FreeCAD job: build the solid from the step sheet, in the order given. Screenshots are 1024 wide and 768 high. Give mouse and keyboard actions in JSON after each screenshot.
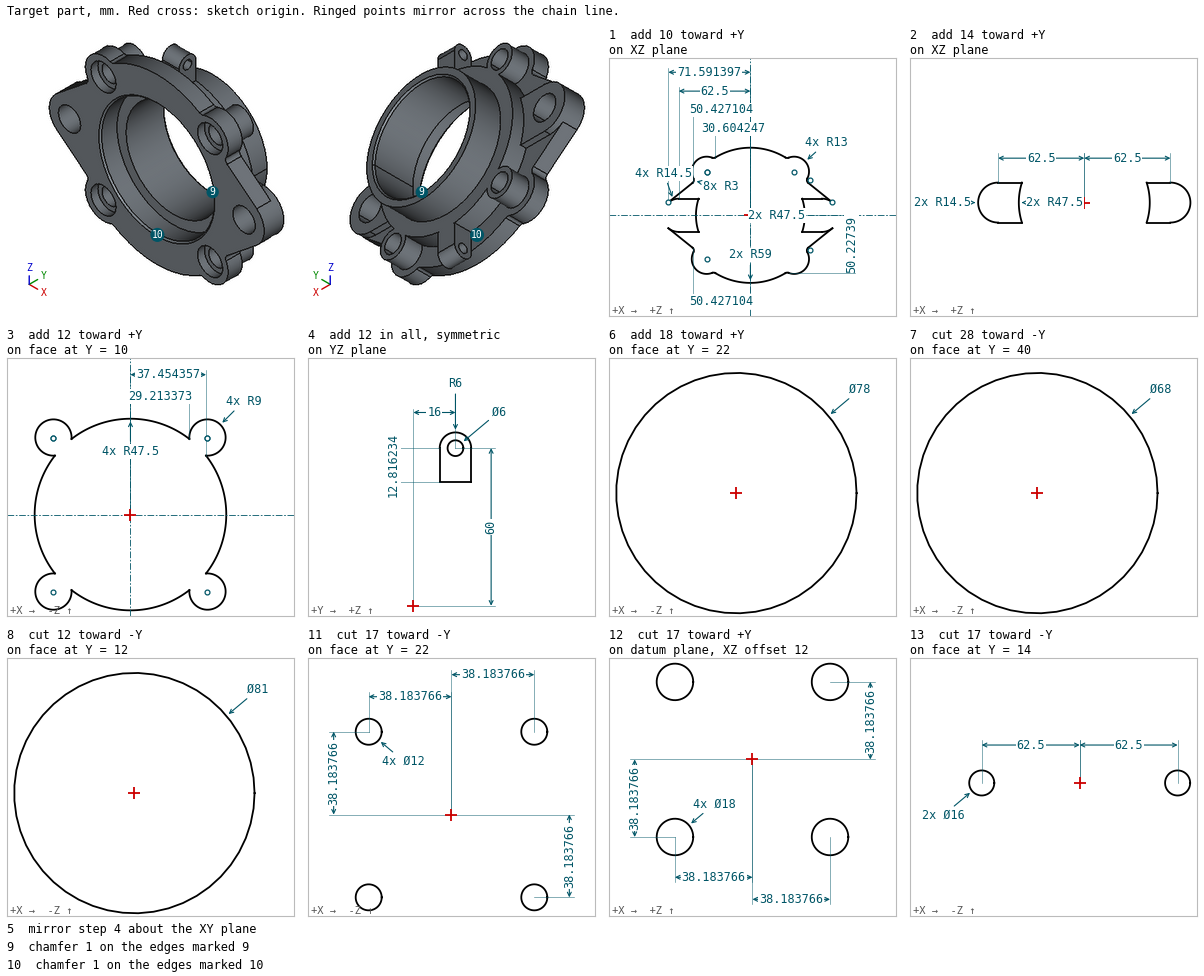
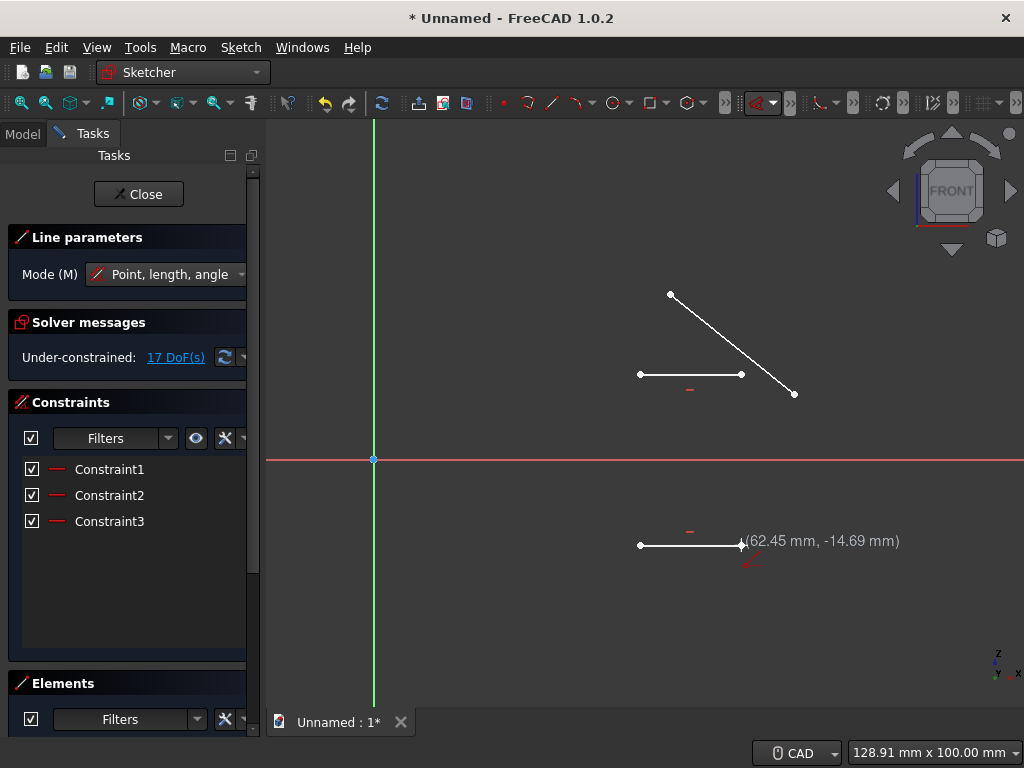
{"action": "left_click", "coordinate": [795, 526]}
{"action": "left_click", "coordinate": [670, 626]}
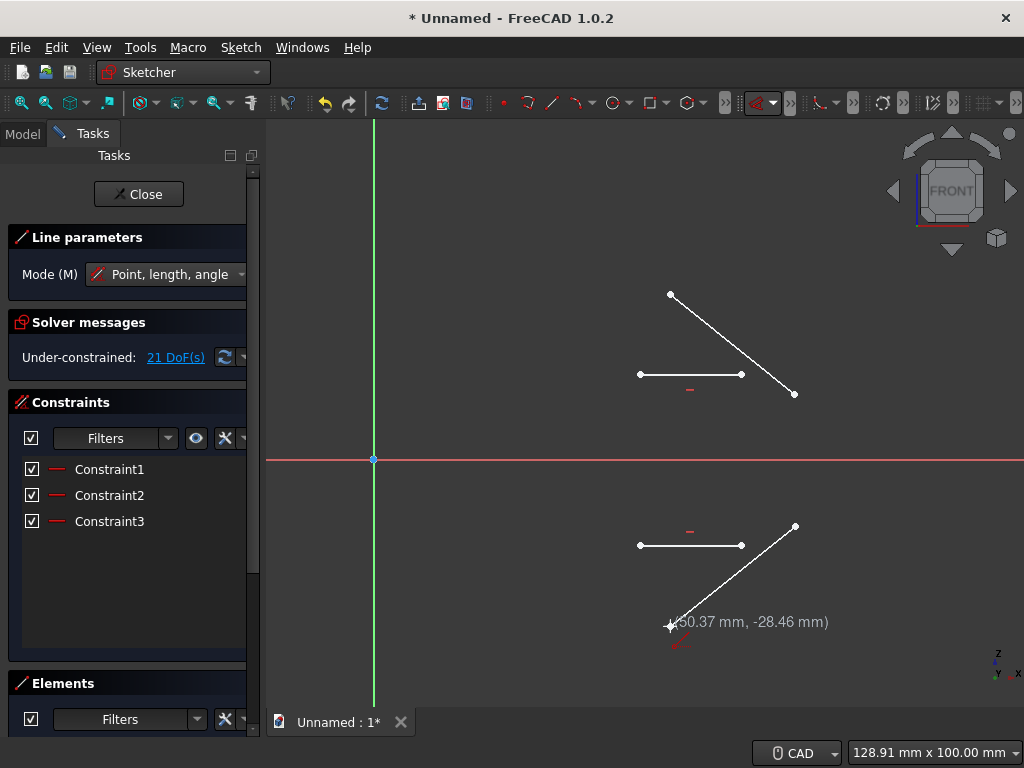
{"action": "scroll", "coordinate": [742, 375], "scroll_direction": "down", "scroll_amount": 4}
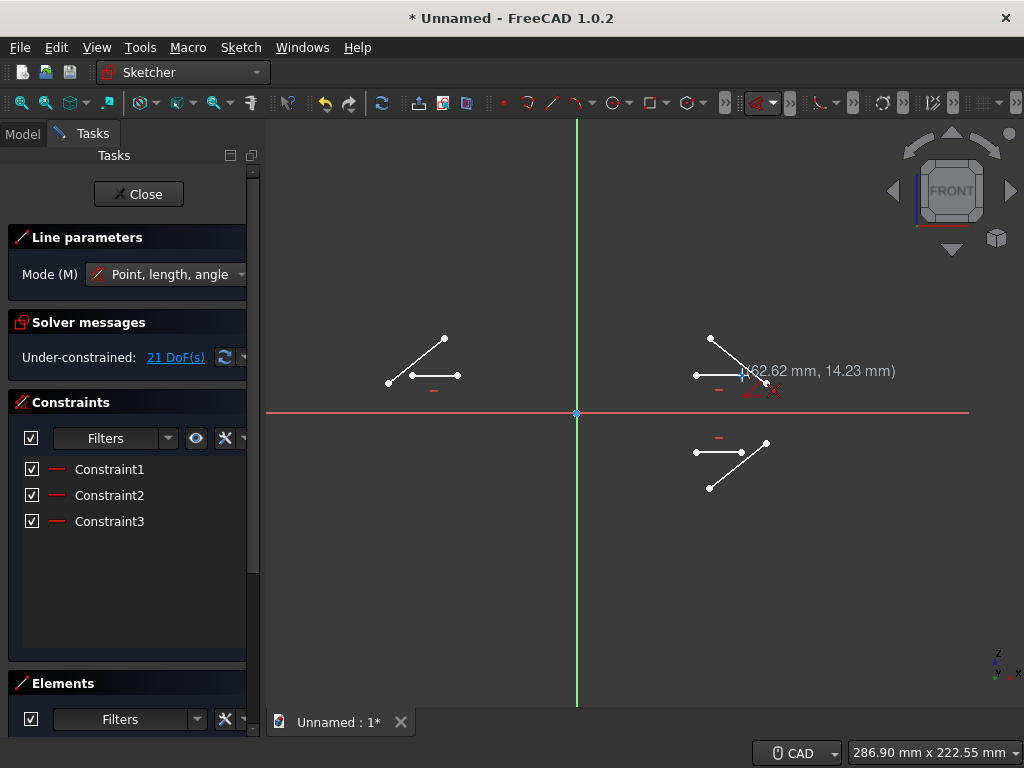
{"action": "left_click", "coordinate": [444, 488]}
{"action": "left_click", "coordinate": [388, 443]}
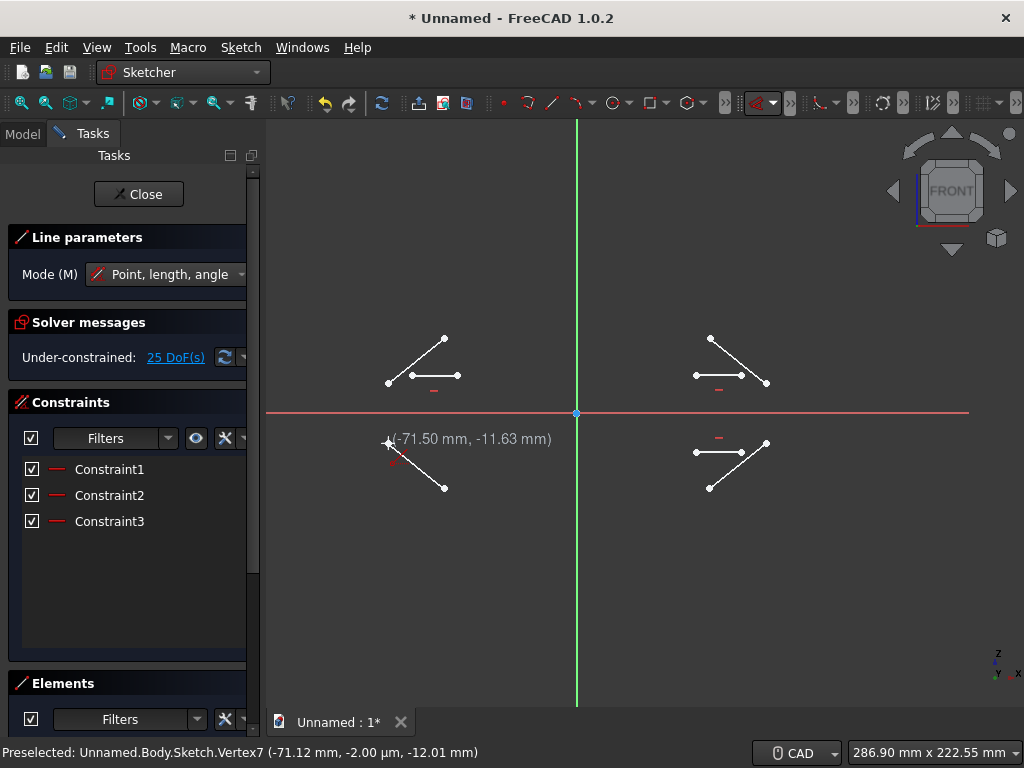
{"action": "scroll", "coordinate": [412, 452], "scroll_direction": "up", "scroll_amount": 4}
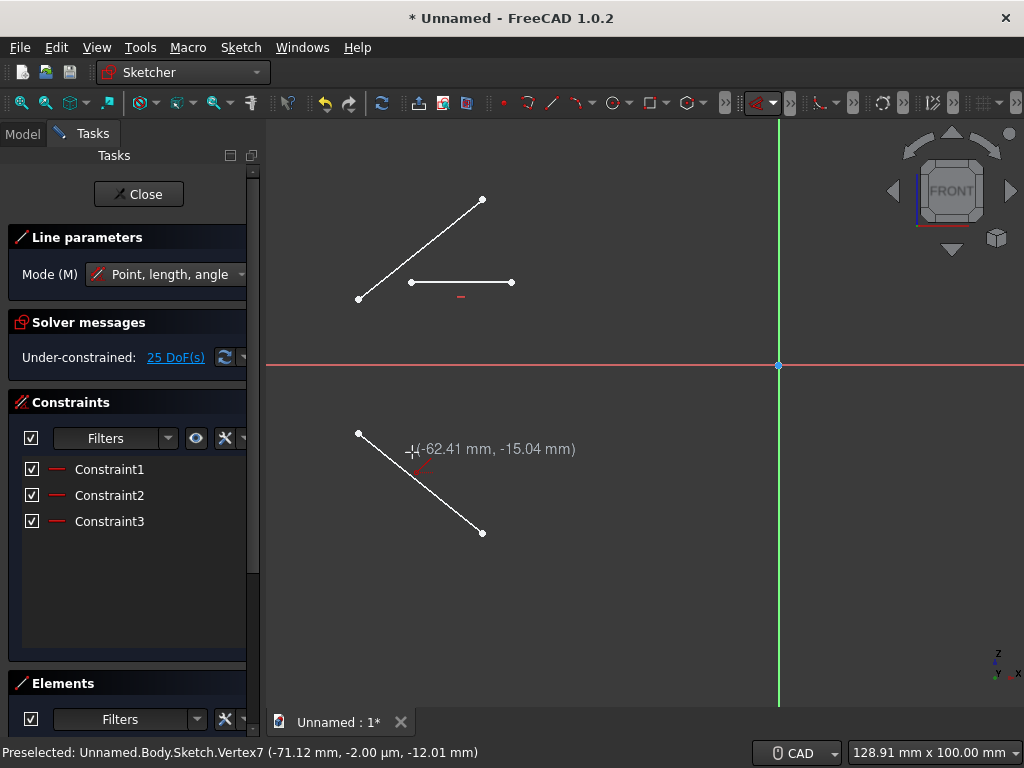
{"action": "left_click", "coordinate": [411, 450]}
{"action": "left_click", "coordinate": [513, 450]}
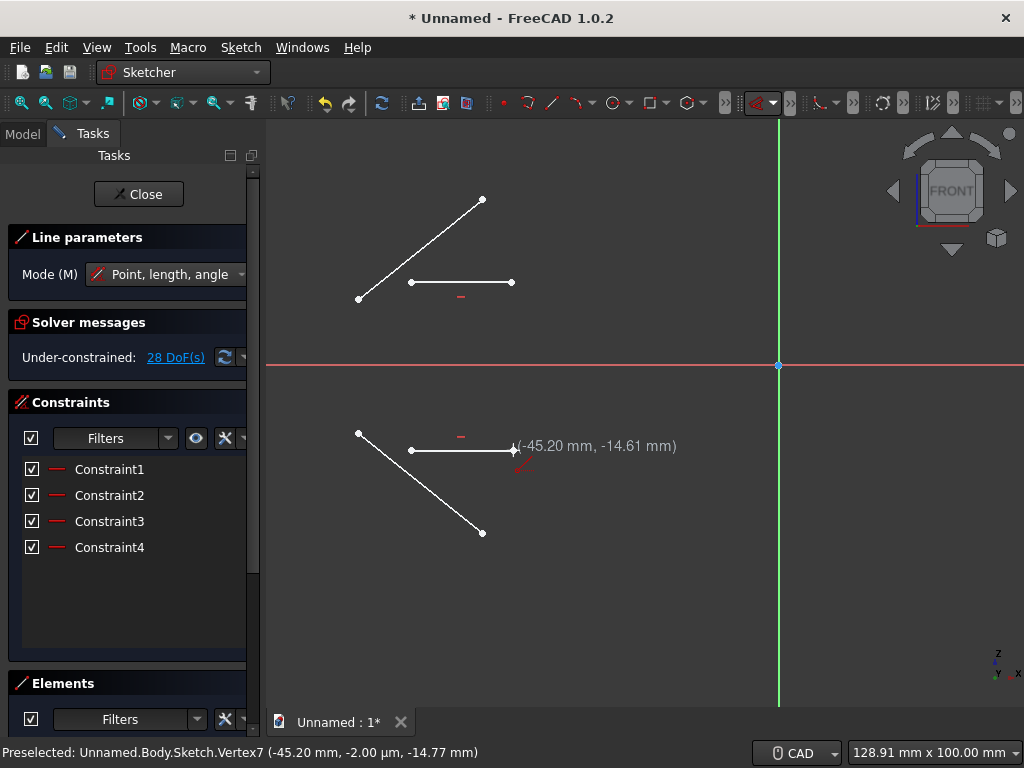
{"action": "key", "text": "g 3 a"}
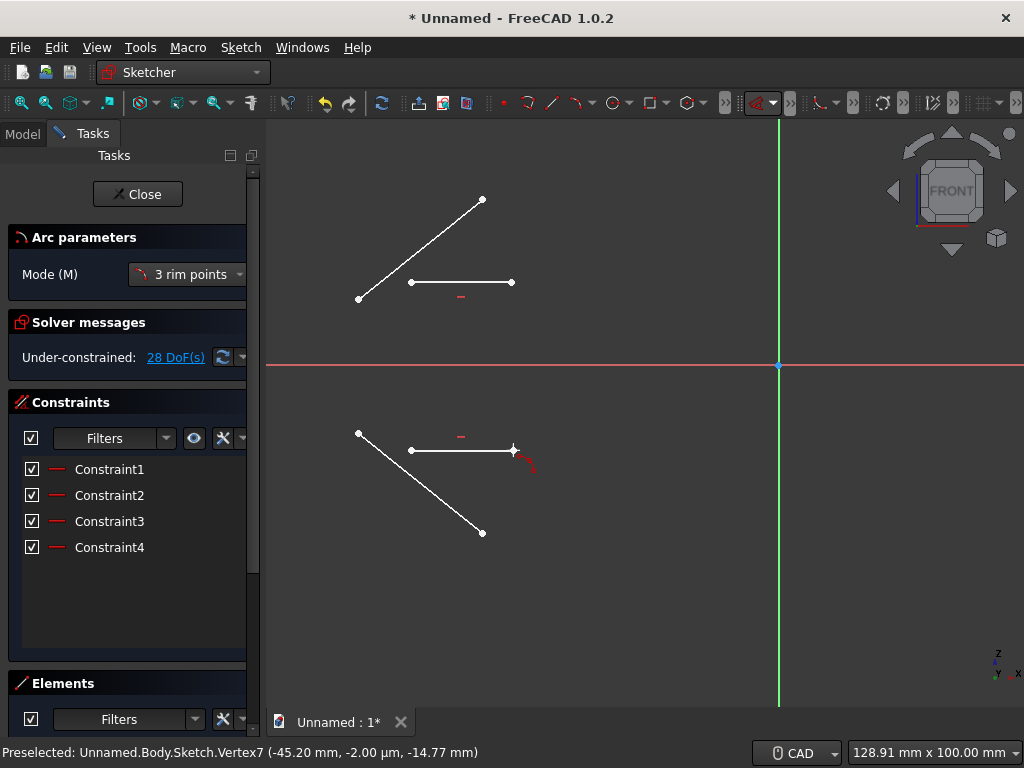
{"action": "left_click", "coordinate": [412, 282]}
{"action": "left_click", "coordinate": [358, 300]}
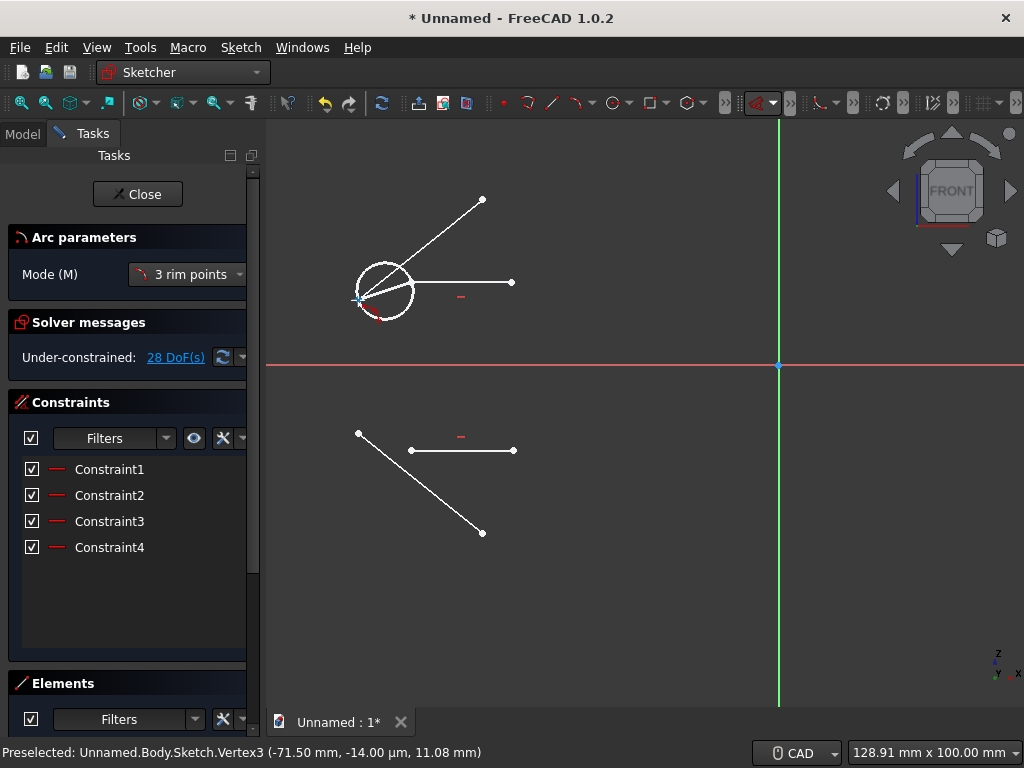
{"action": "scroll", "coordinate": [383, 285], "scroll_direction": "up", "scroll_amount": 6}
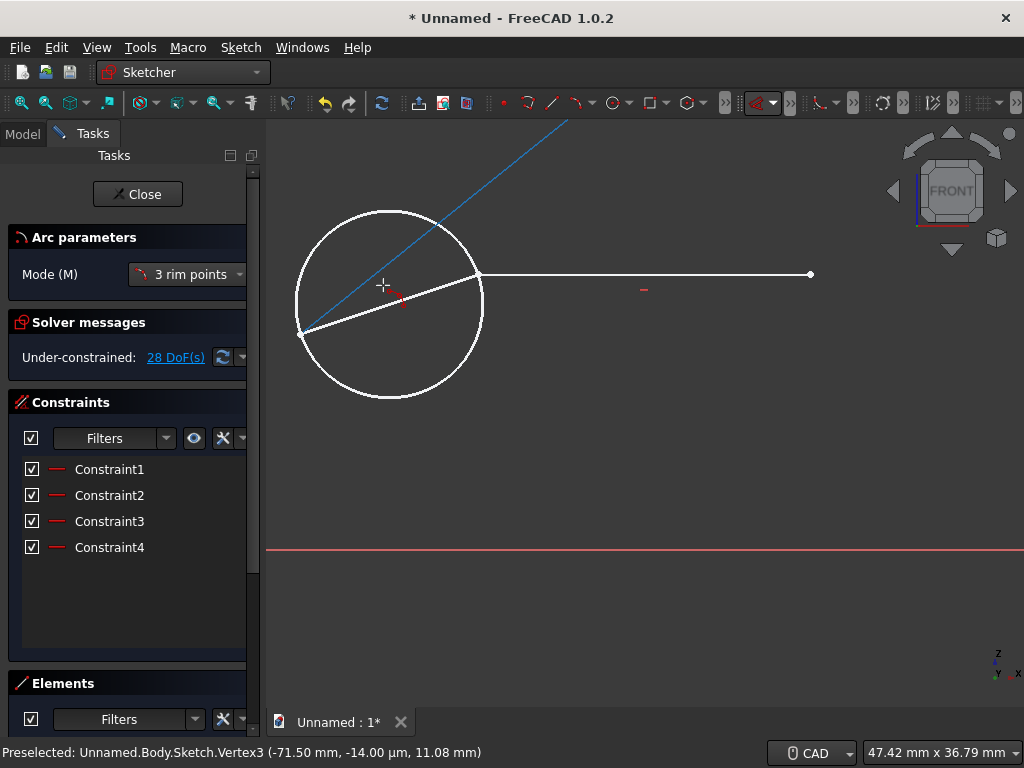
{"action": "left_click", "coordinate": [382, 283]}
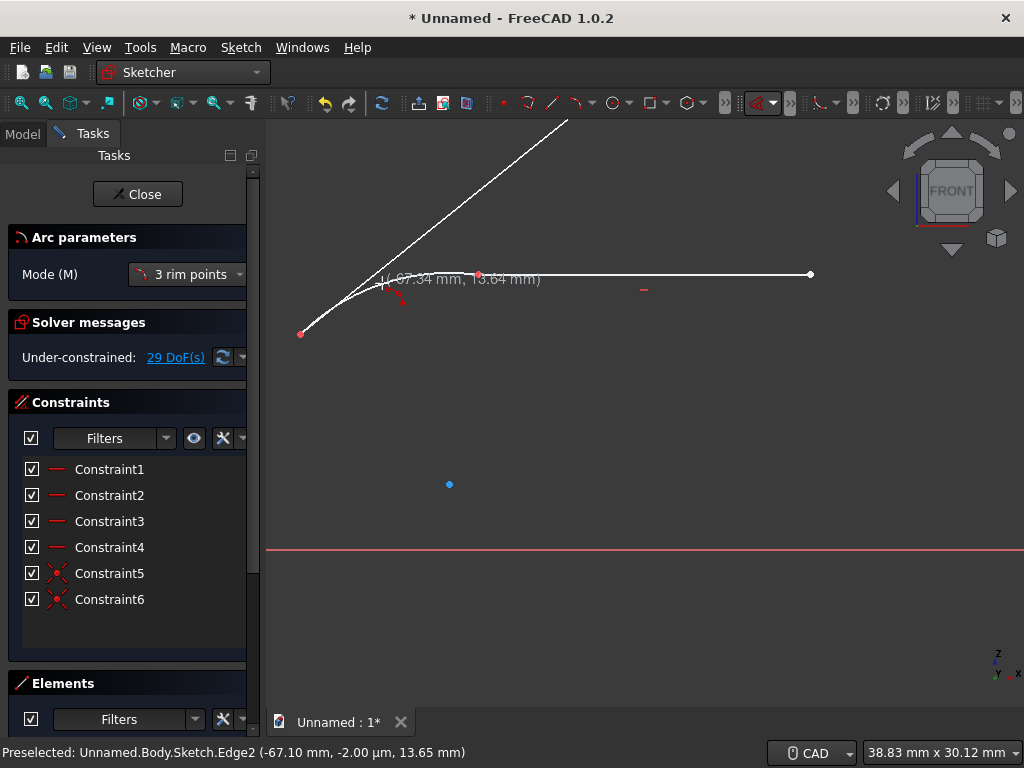
{"action": "scroll", "coordinate": [401, 392], "scroll_direction": "down", "scroll_amount": 10}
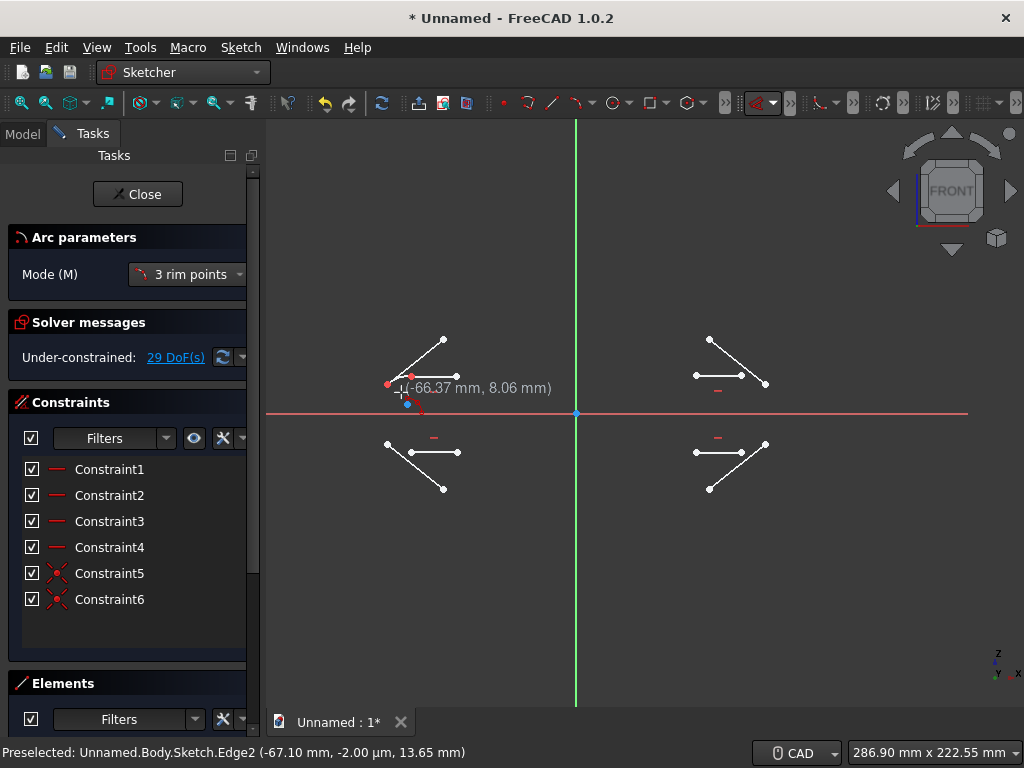
{"action": "left_click", "coordinate": [444, 340]}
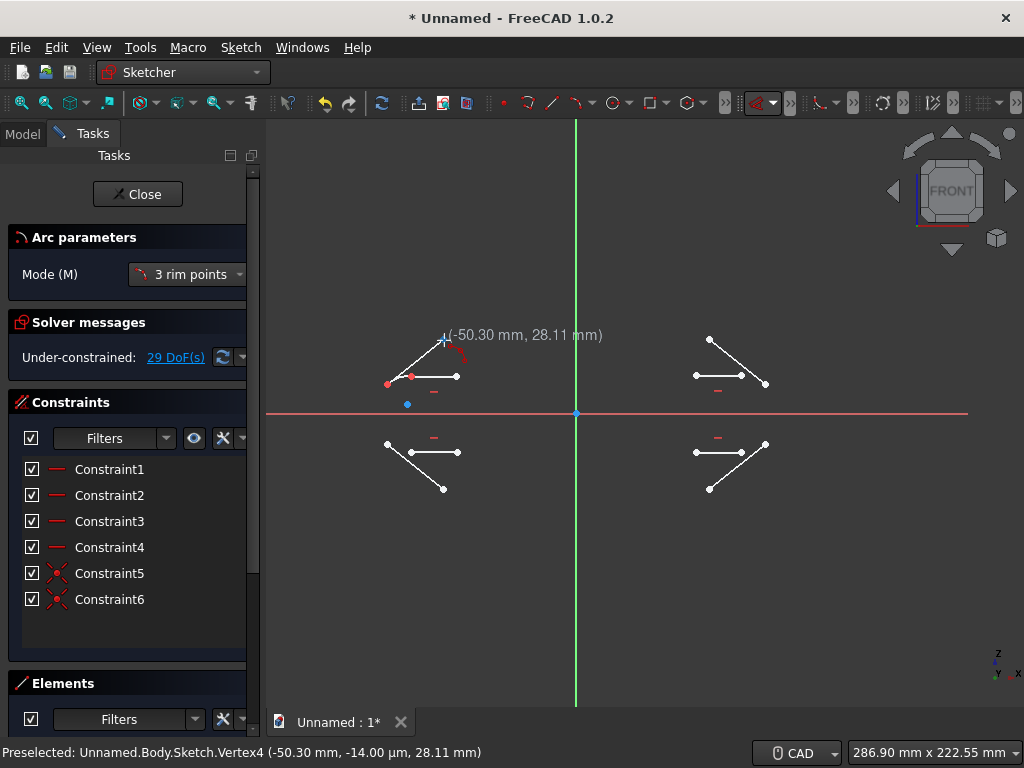
{"action": "scroll", "coordinate": [445, 329], "scroll_direction": "up", "scroll_amount": 3}